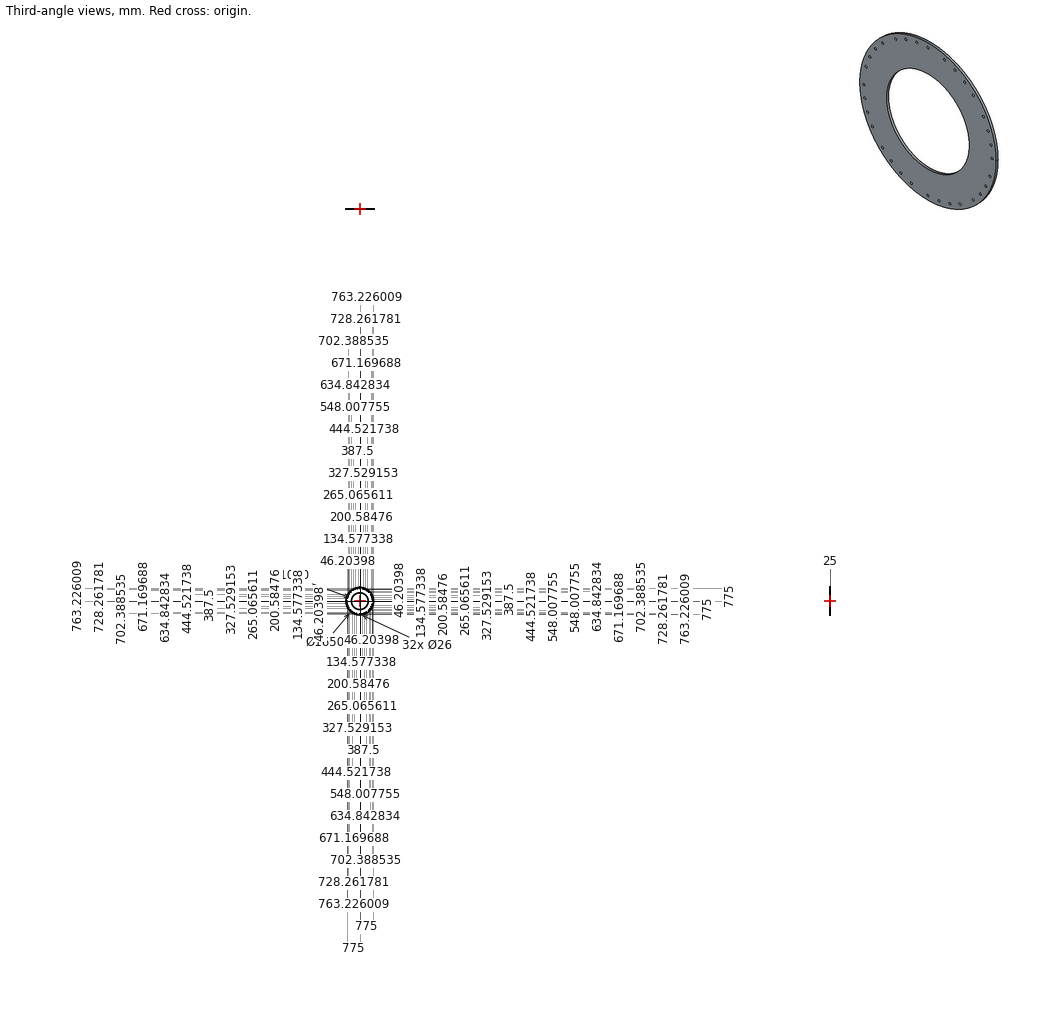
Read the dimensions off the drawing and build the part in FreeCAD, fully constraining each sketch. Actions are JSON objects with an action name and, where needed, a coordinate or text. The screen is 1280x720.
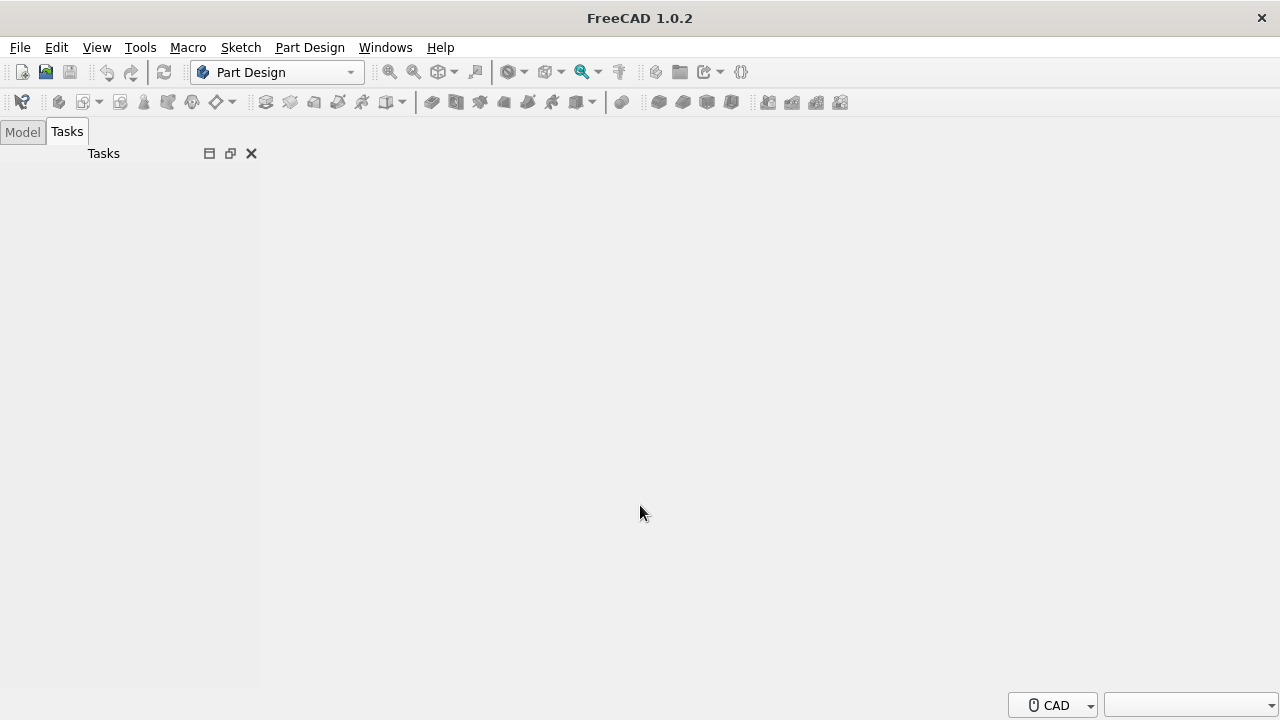
{"action": "key", "text": "ctrl+n"}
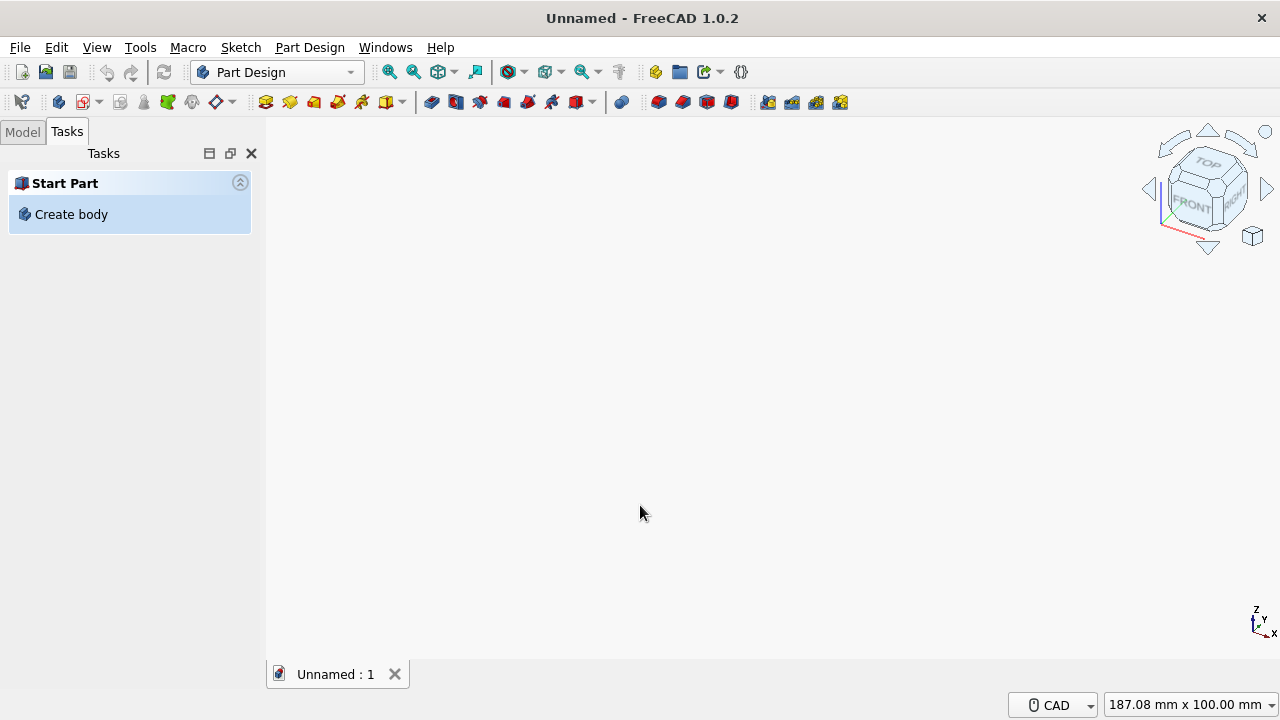
{"action": "left_click", "coordinate": [84, 102]}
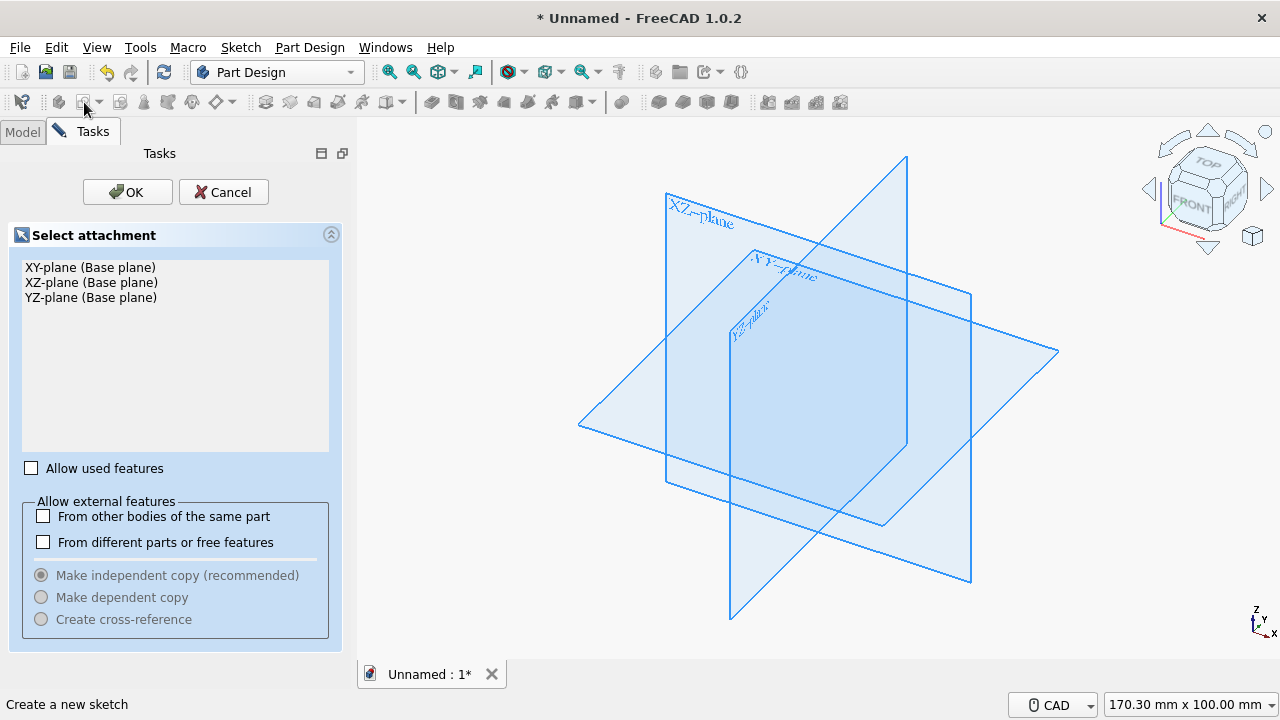
{"action": "left_click", "coordinate": [82, 282]}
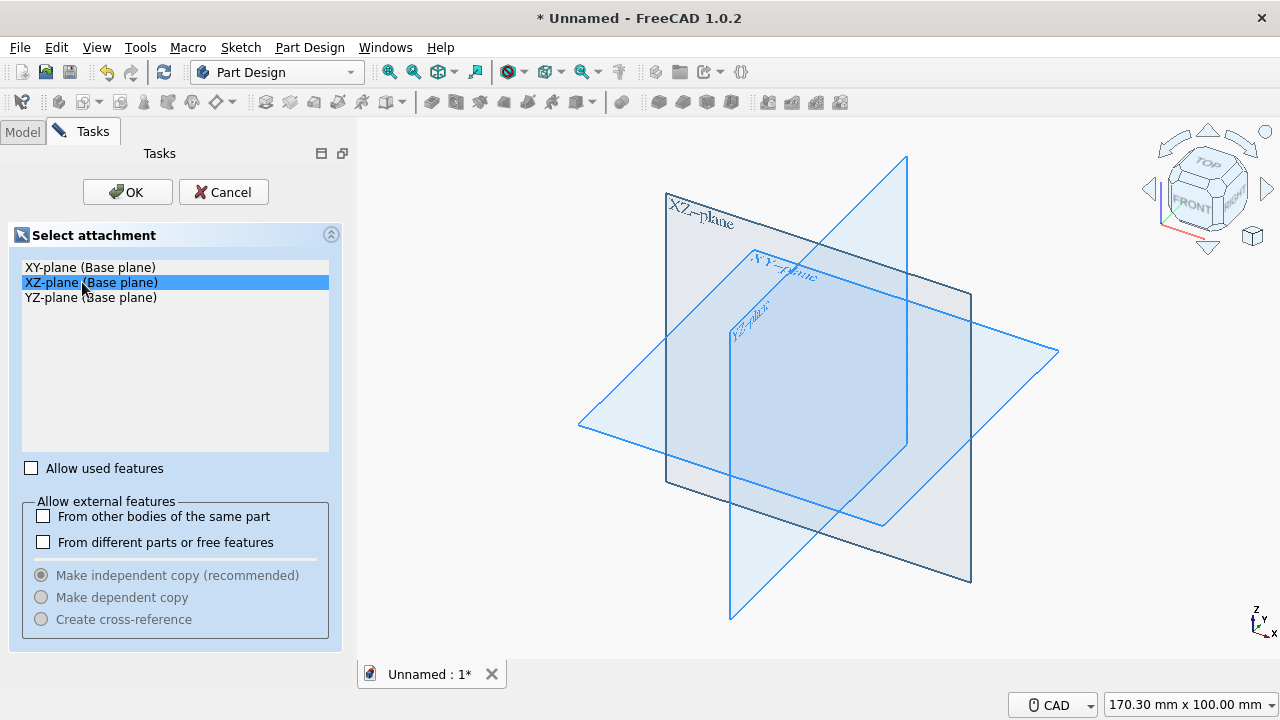
{"action": "left_click", "coordinate": [128, 192]}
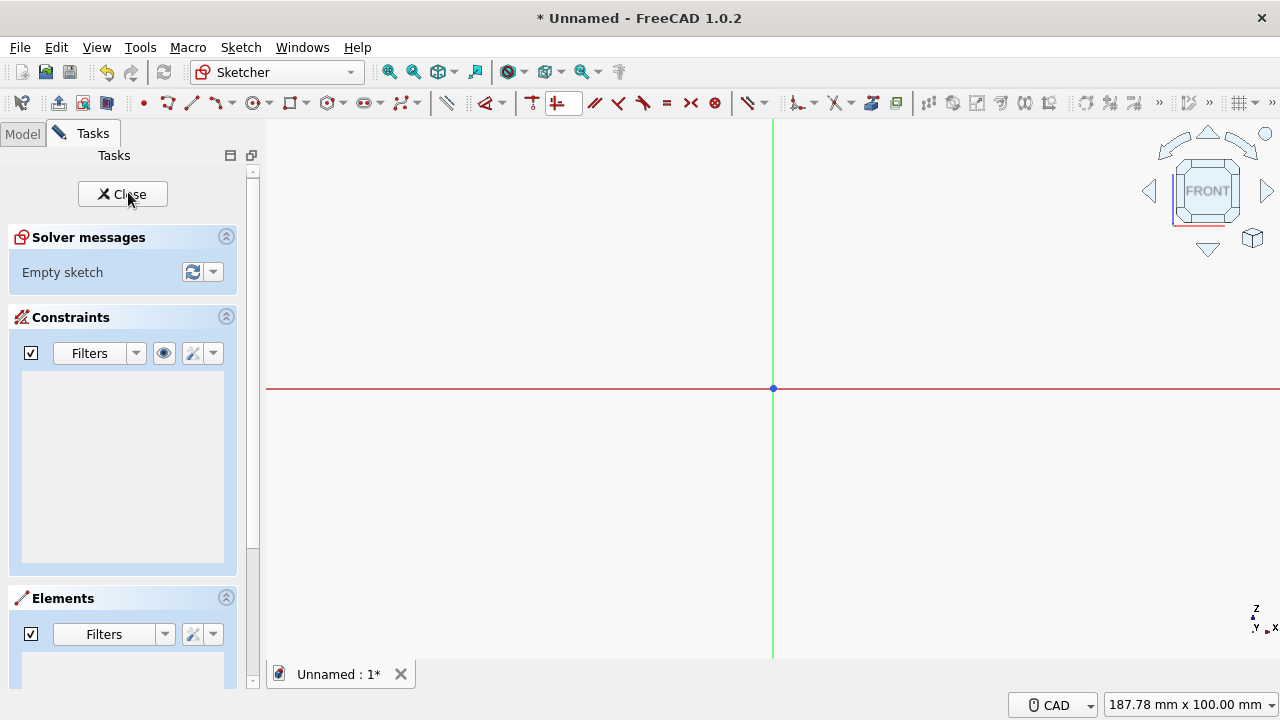
{"action": "scroll", "coordinate": [702, 389], "scroll_direction": "down", "scroll_amount": 16}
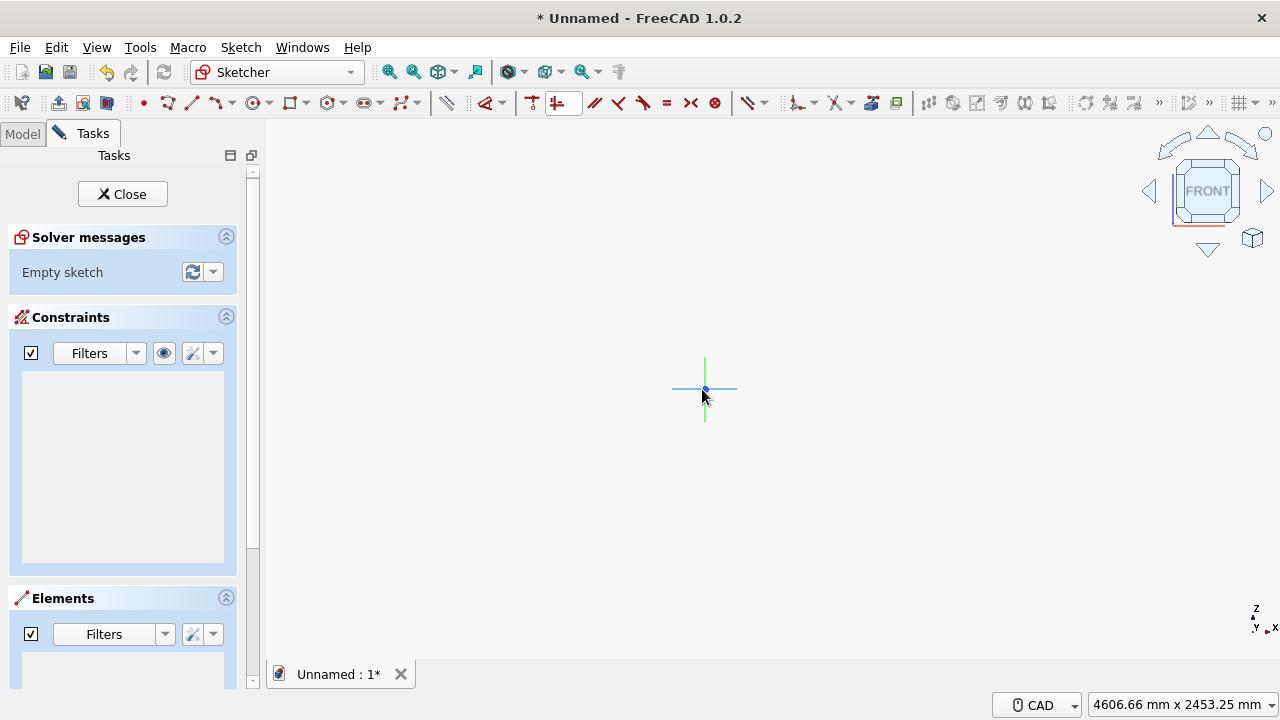
{"action": "left_click", "coordinate": [254, 104]}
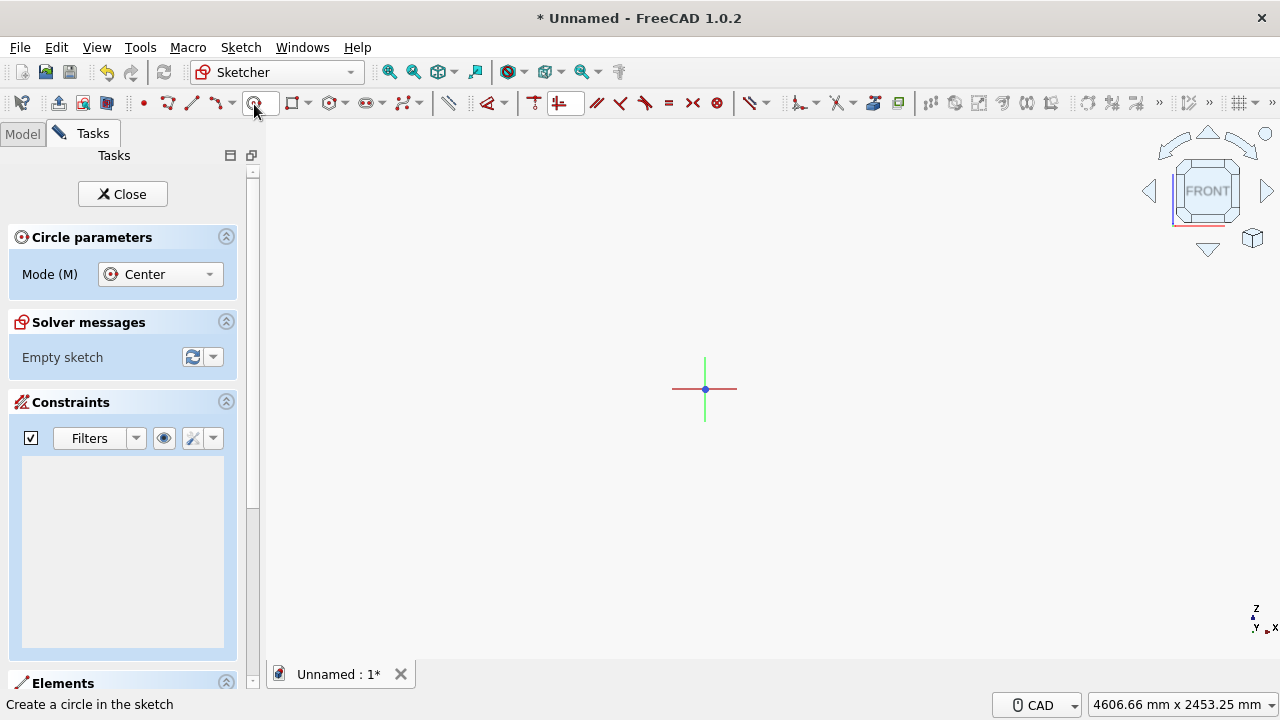
{"action": "left_click", "coordinate": [705, 389]}
{"action": "left_click", "coordinate": [834, 261]}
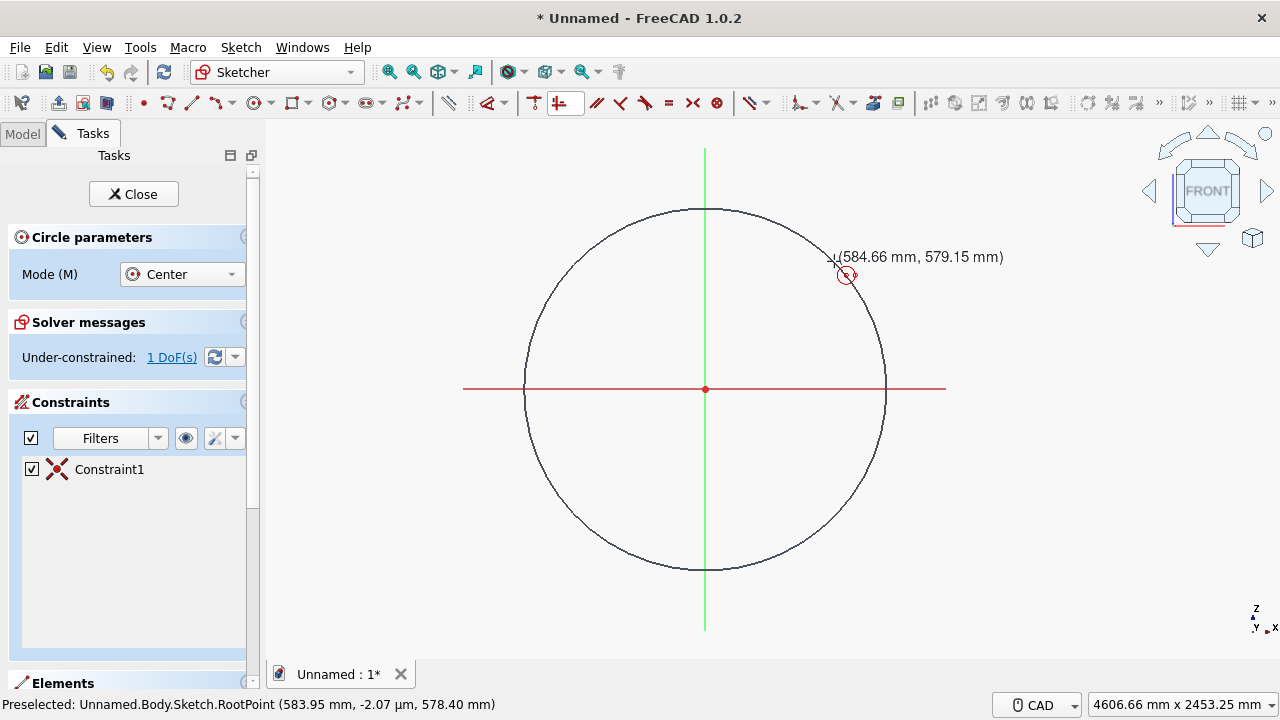
{"action": "left_click", "coordinate": [705, 389]}
{"action": "left_click", "coordinate": [783, 312]}
{"action": "key", "text": "Escape"}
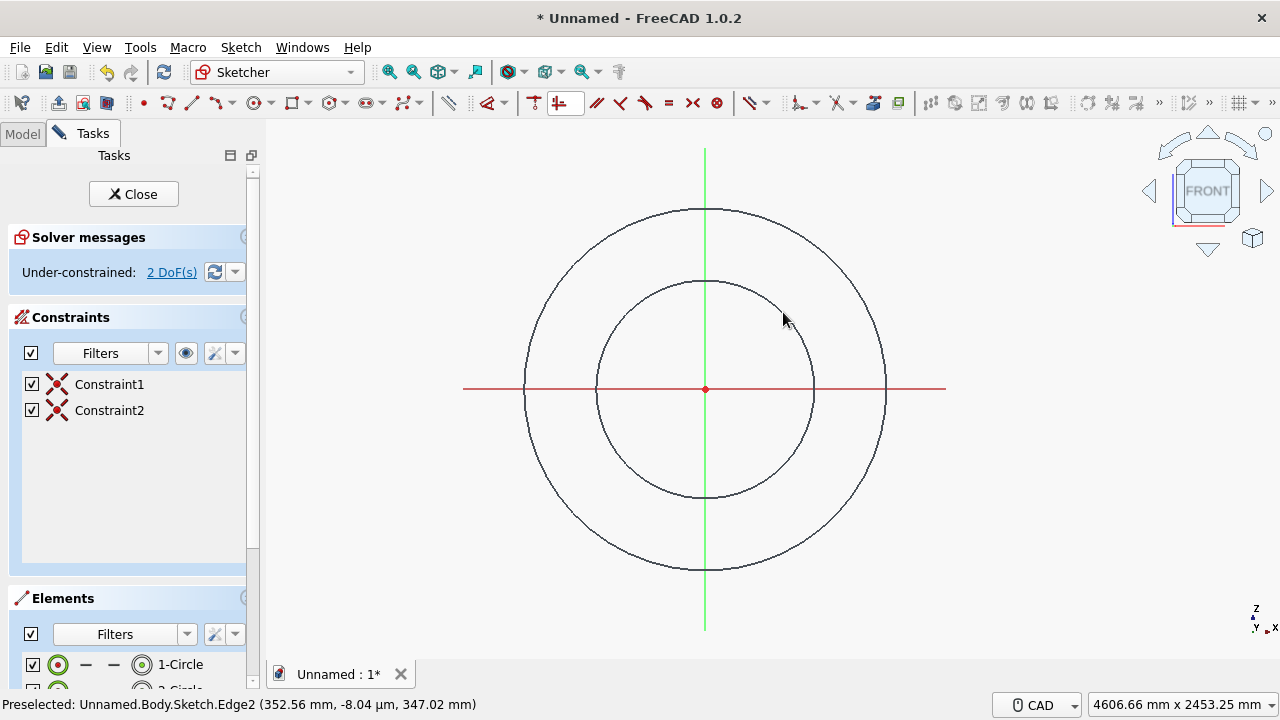
{"action": "left_click", "coordinate": [833, 261]}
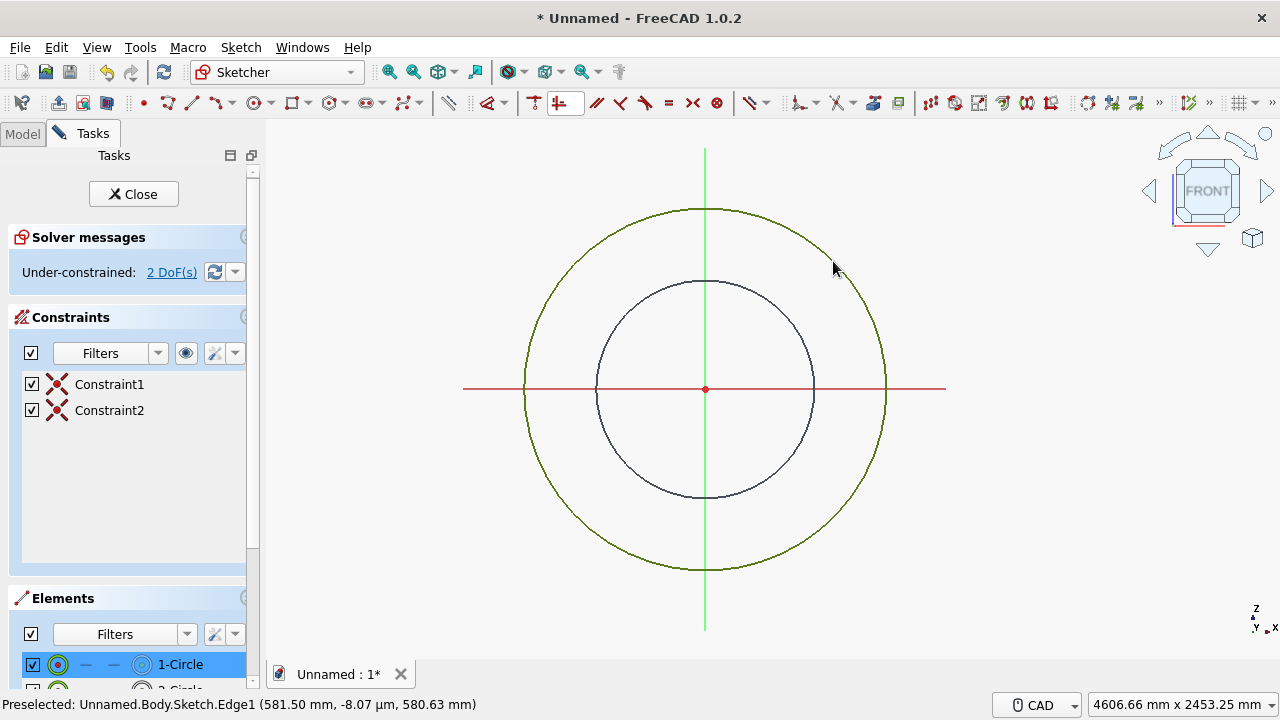
{"action": "key", "text": "k o"}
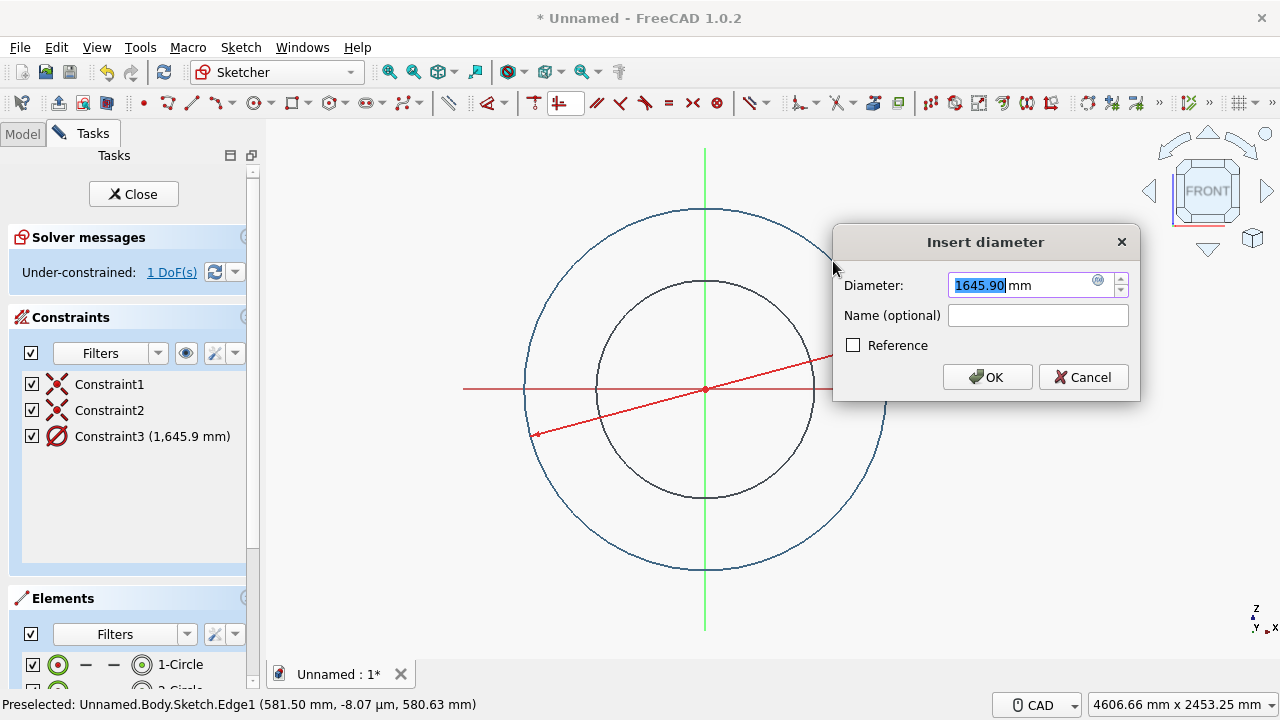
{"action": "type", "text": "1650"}
{"action": "key", "text": "Return"}